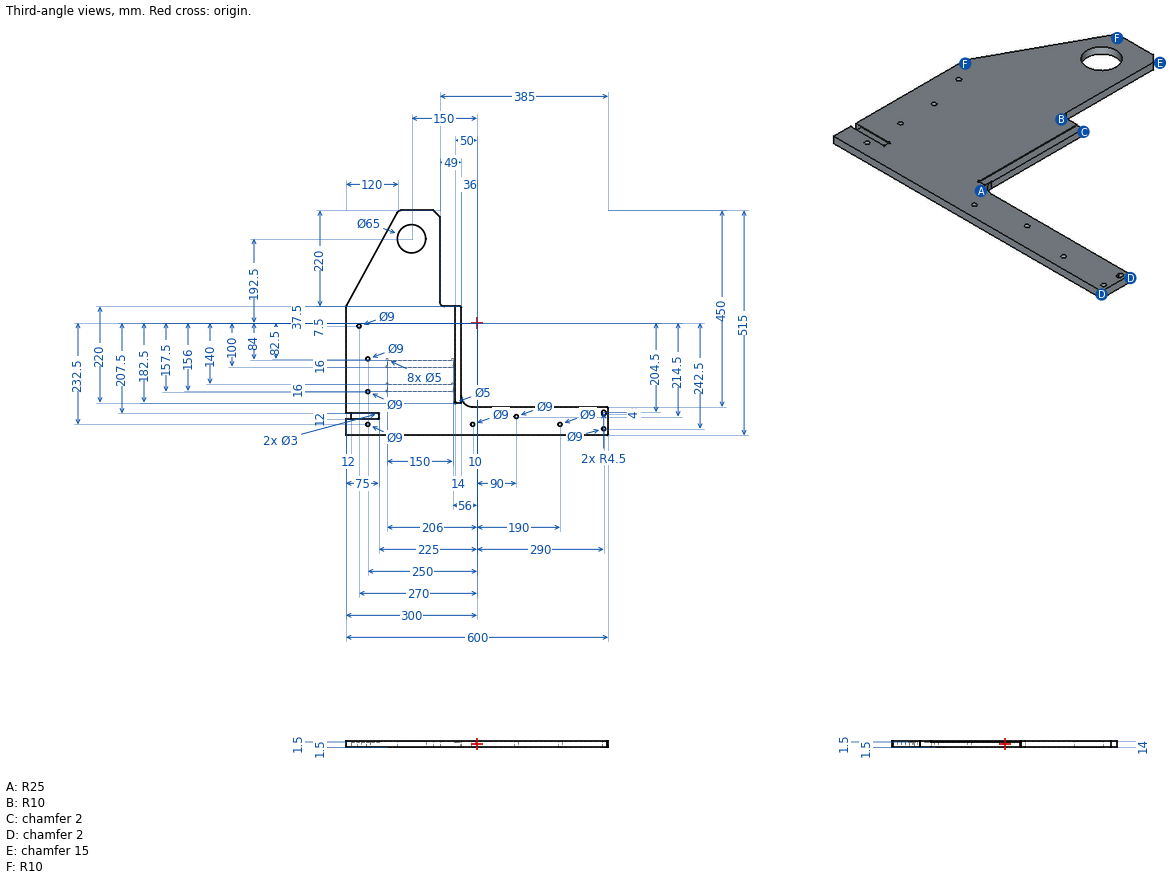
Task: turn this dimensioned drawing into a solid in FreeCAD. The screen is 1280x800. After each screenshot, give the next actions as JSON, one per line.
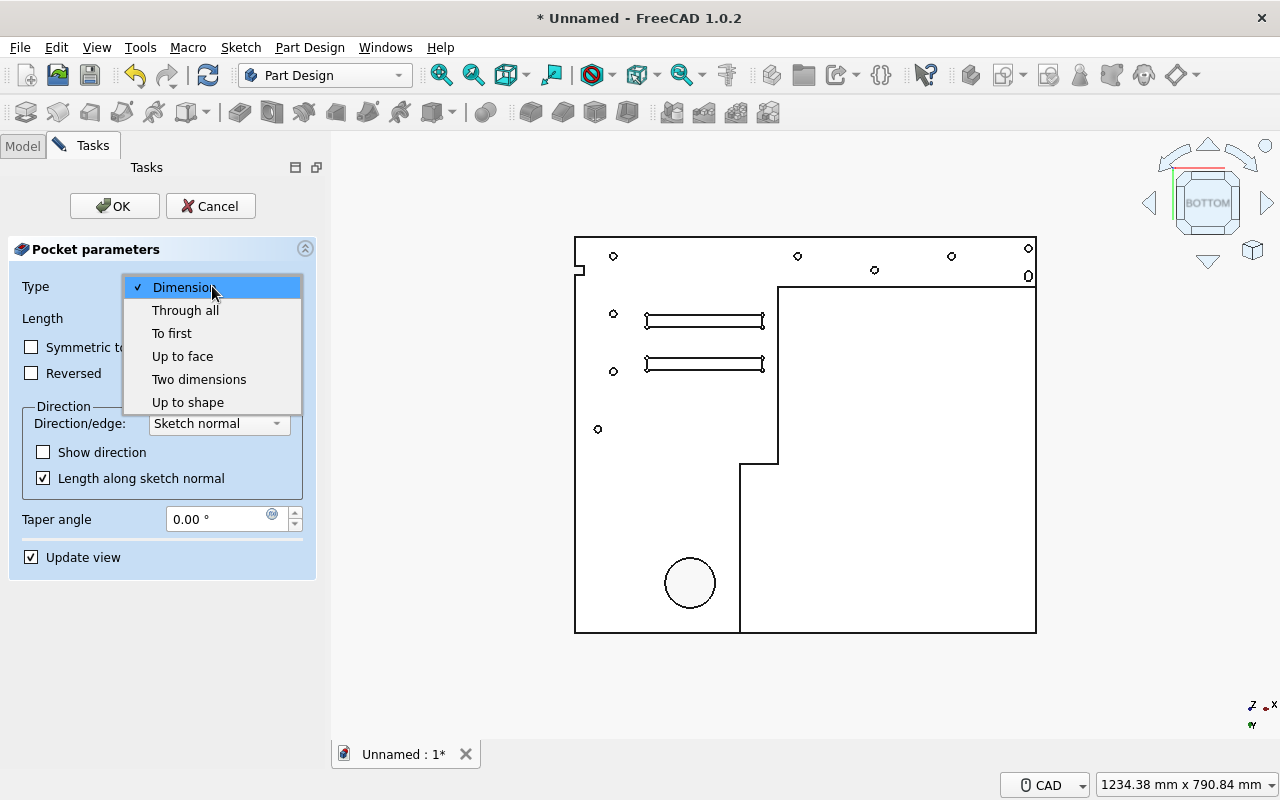
{"action": "left_click", "coordinate": [212, 334]}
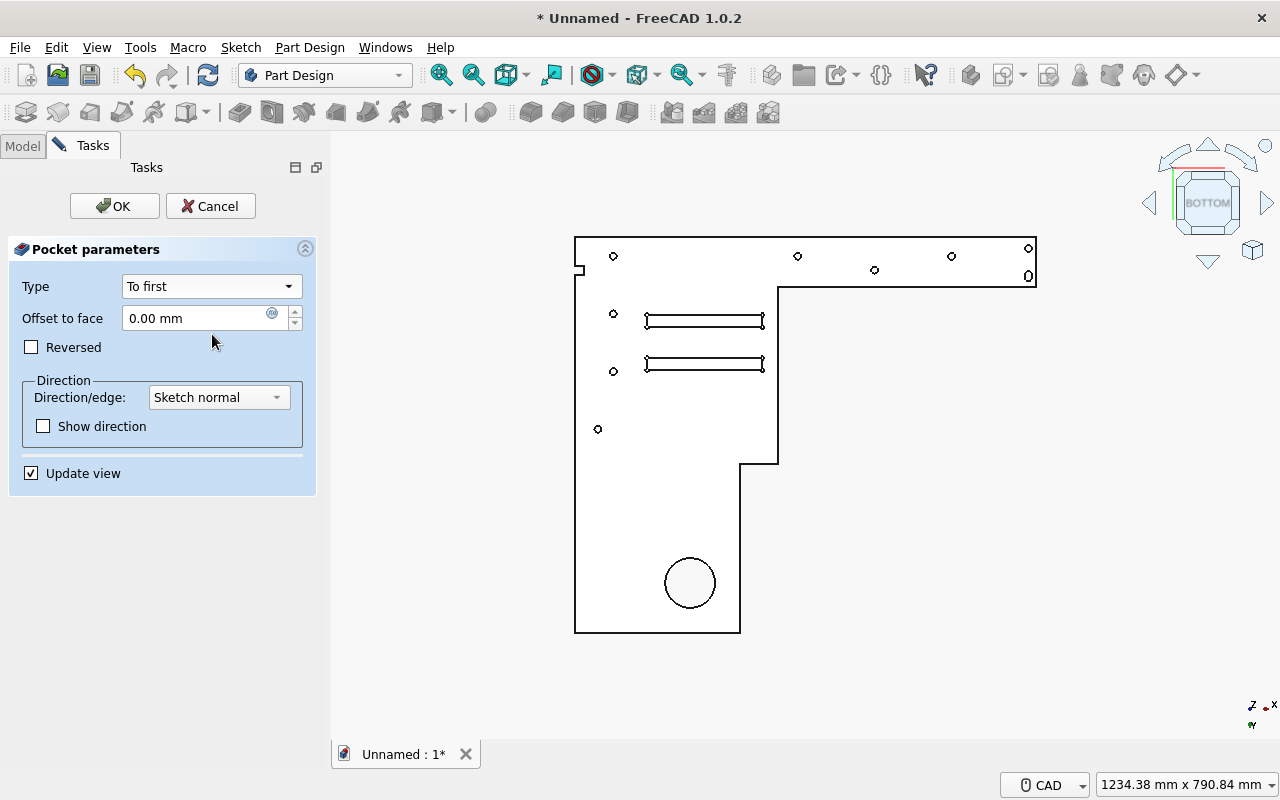
{"action": "left_click", "coordinate": [115, 206]}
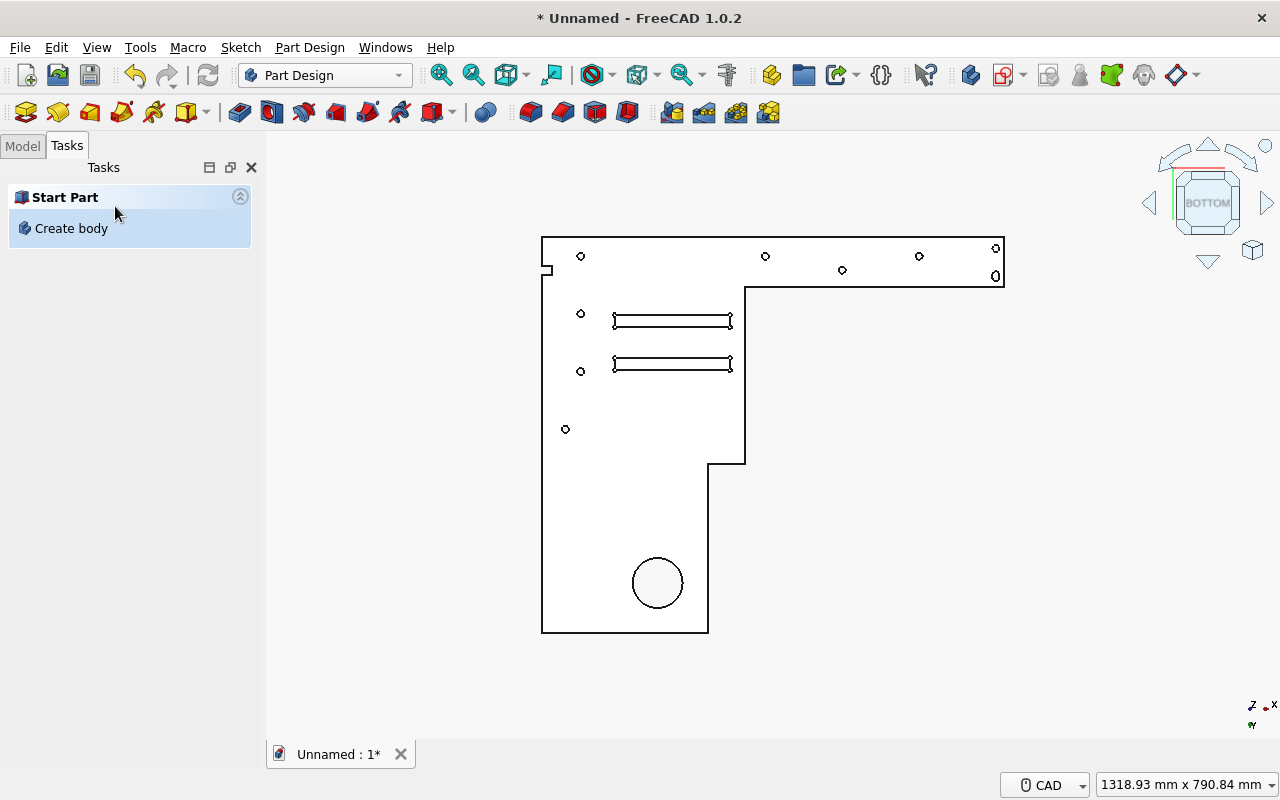
{"action": "scroll", "coordinate": [745, 286], "scroll_direction": "up", "scroll_amount": 7}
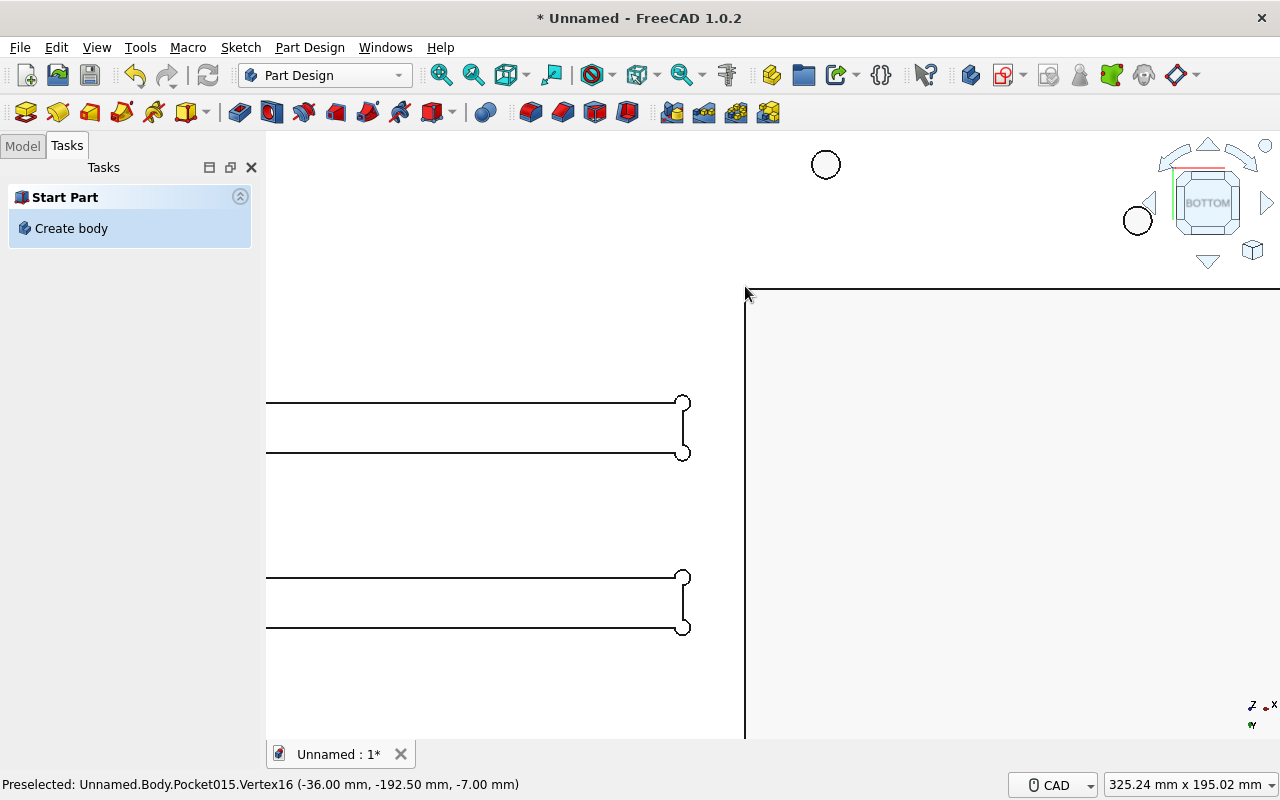
{"action": "left_click", "coordinate": [442, 76]}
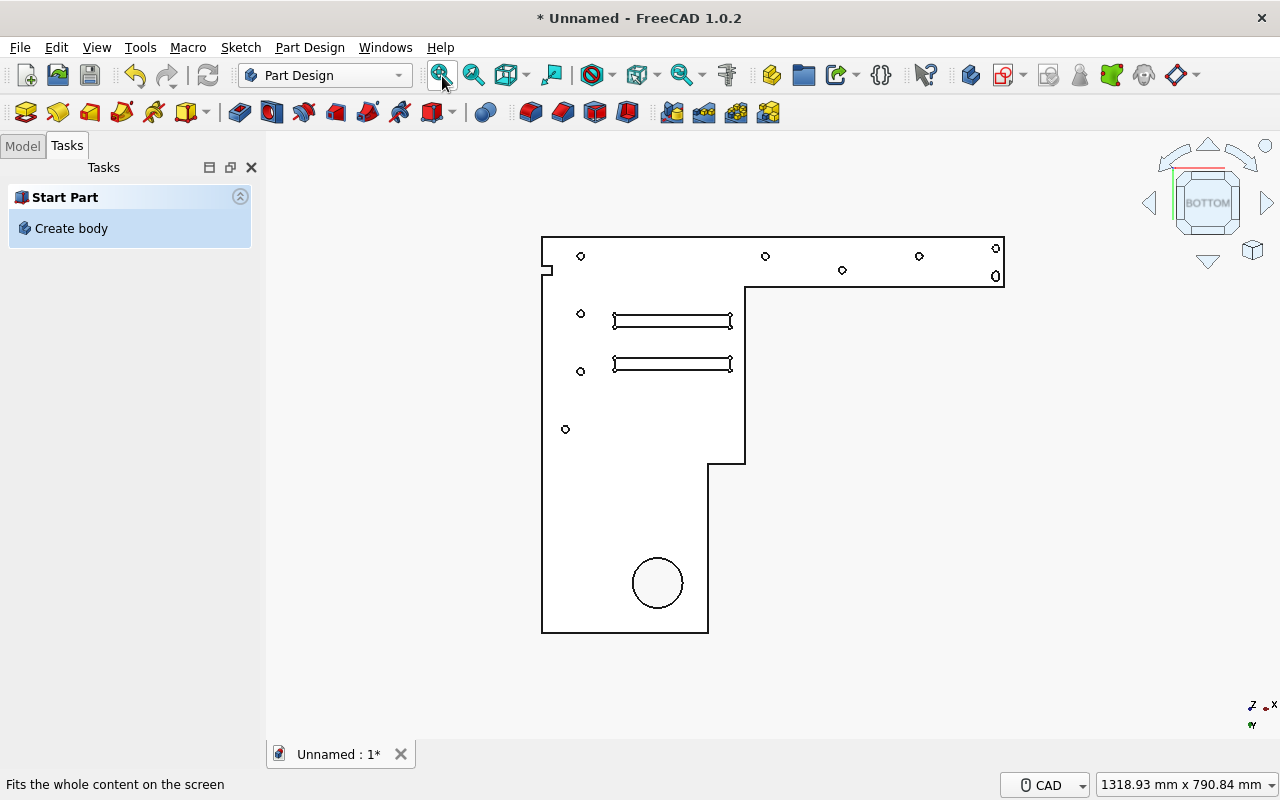
{"action": "key", "text": "0"}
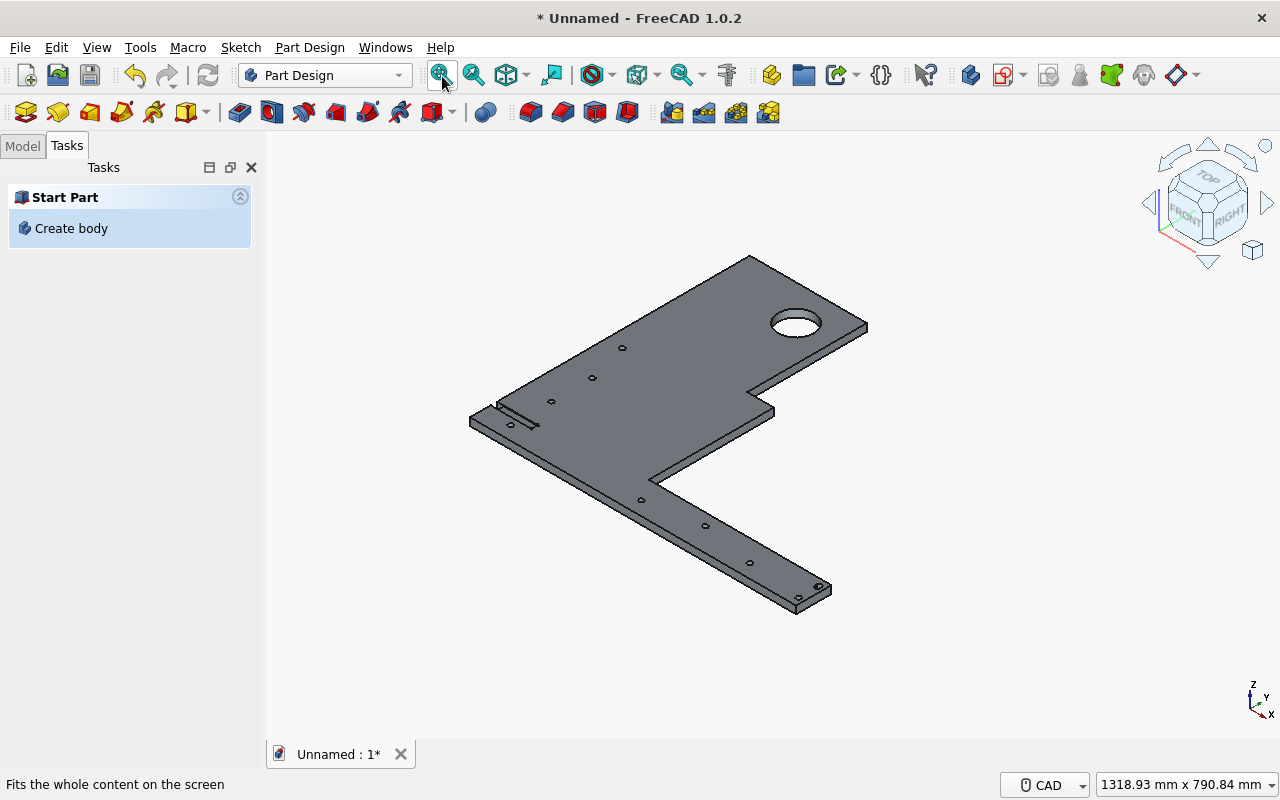
{"action": "scroll", "coordinate": [649, 483], "scroll_direction": "up", "scroll_amount": 7}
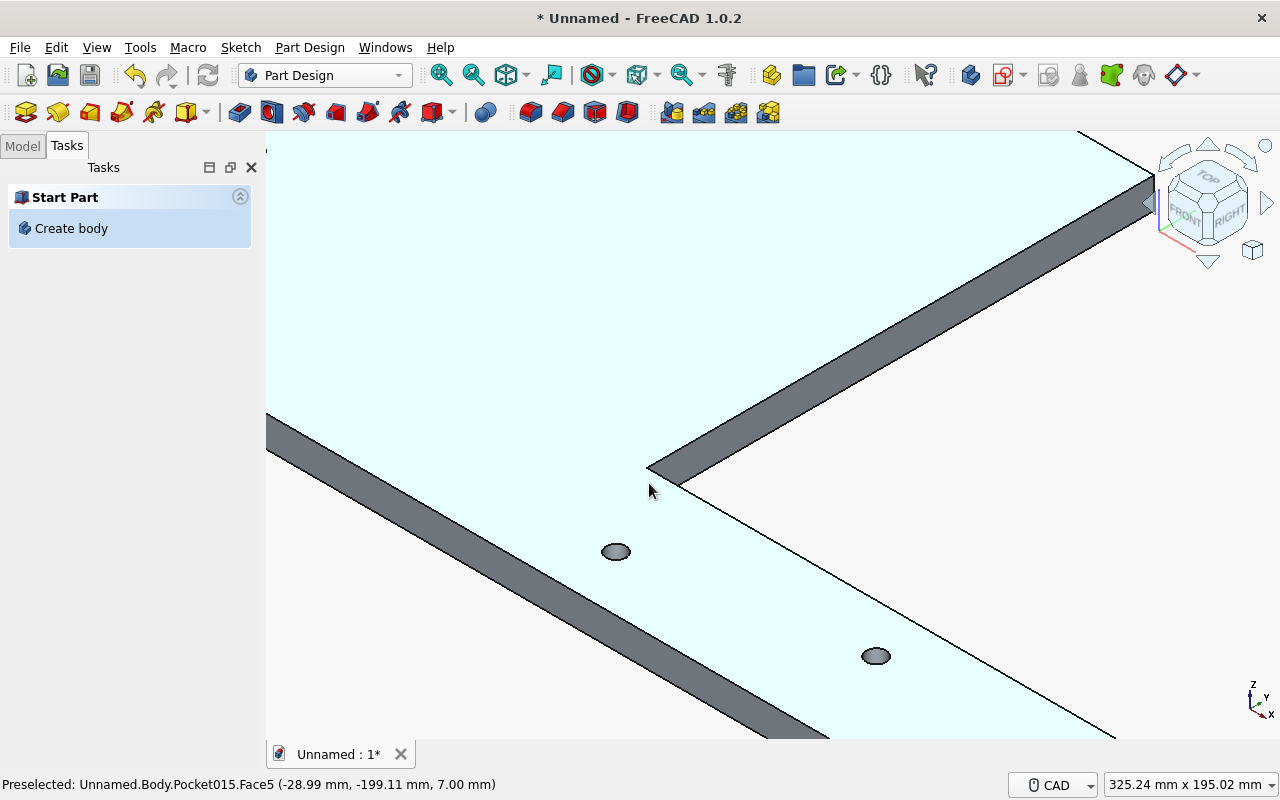
{"action": "left_click", "coordinate": [442, 76]}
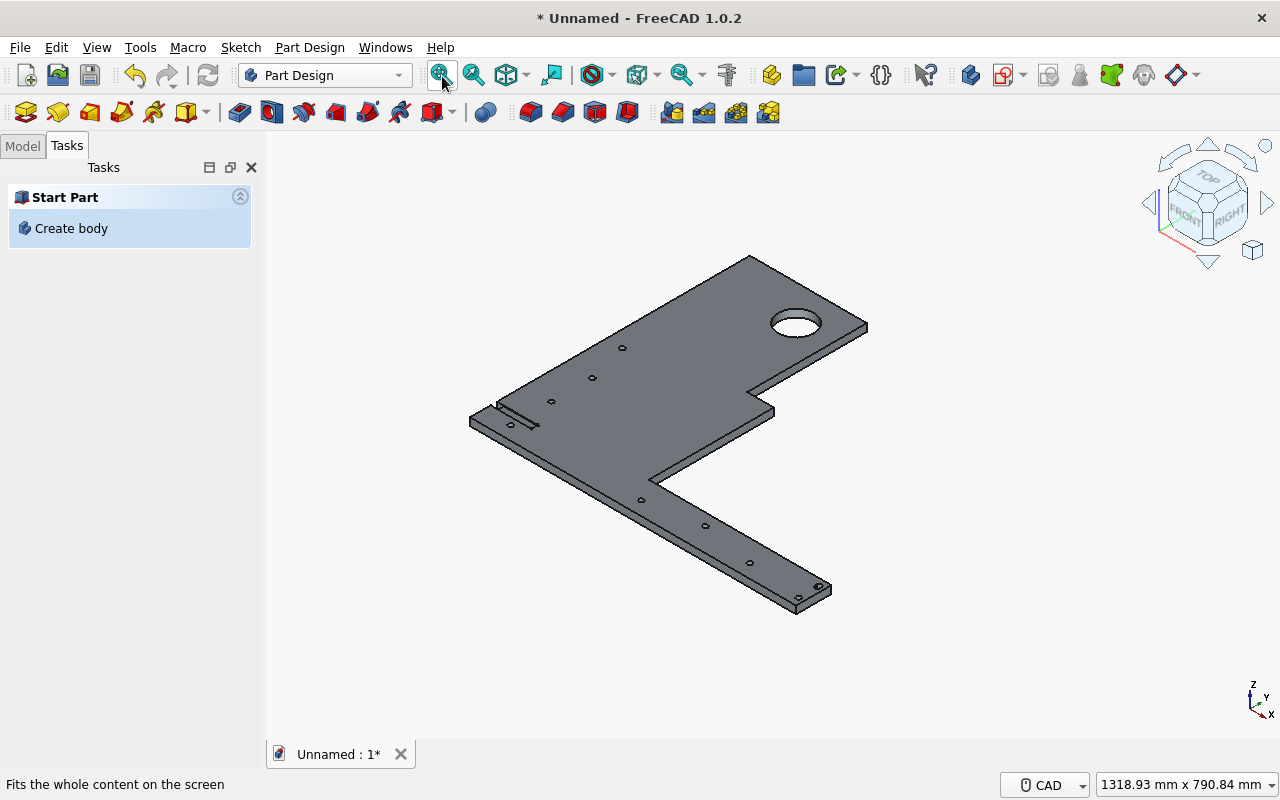
{"action": "key", "text": "2"}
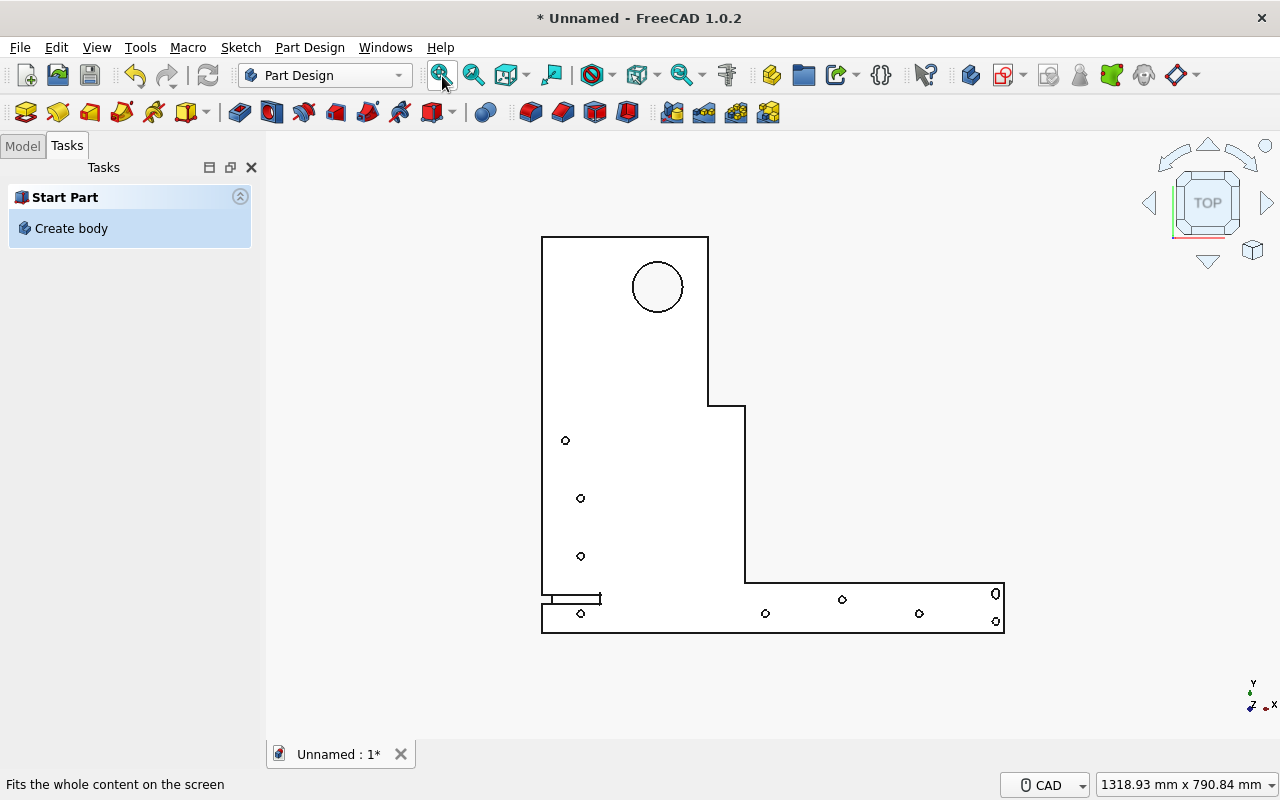
{"action": "scroll", "coordinate": [745, 582], "scroll_direction": "up", "scroll_amount": 7}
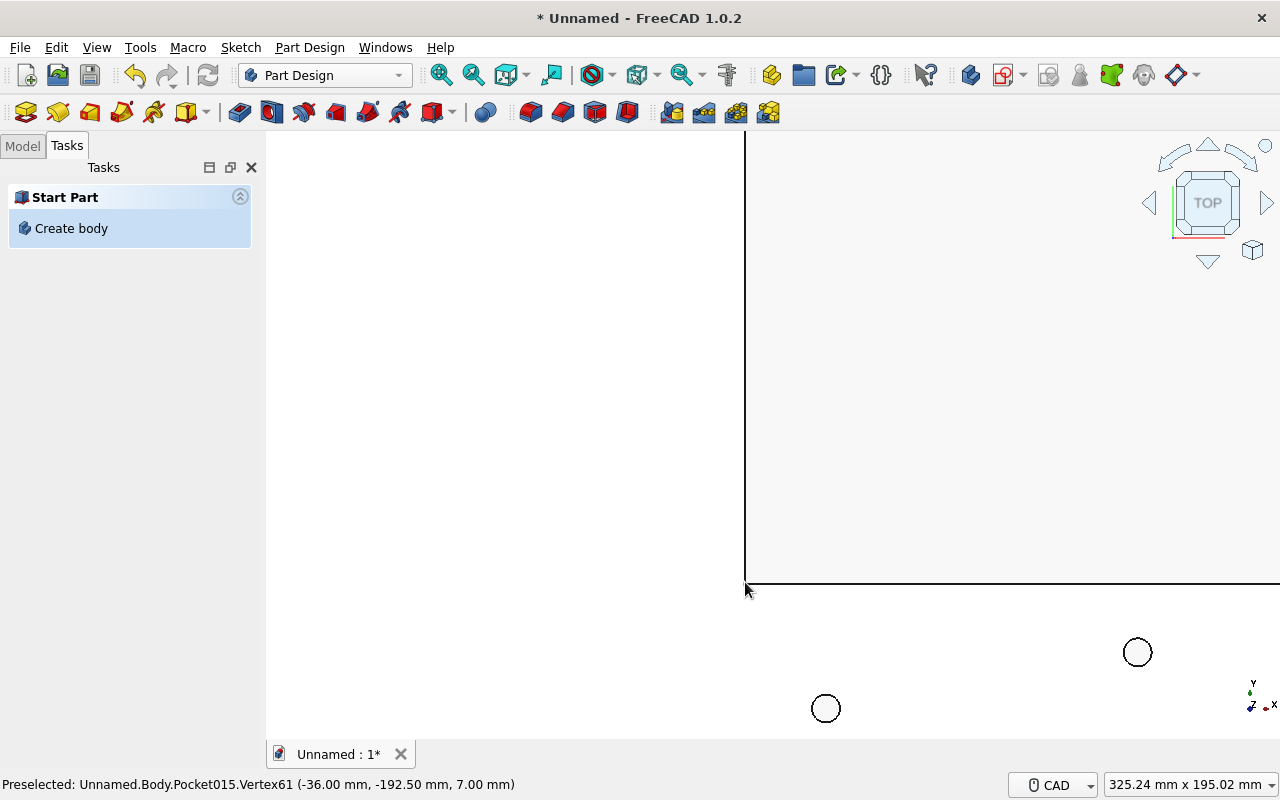
{"action": "left_click", "coordinate": [442, 76]}